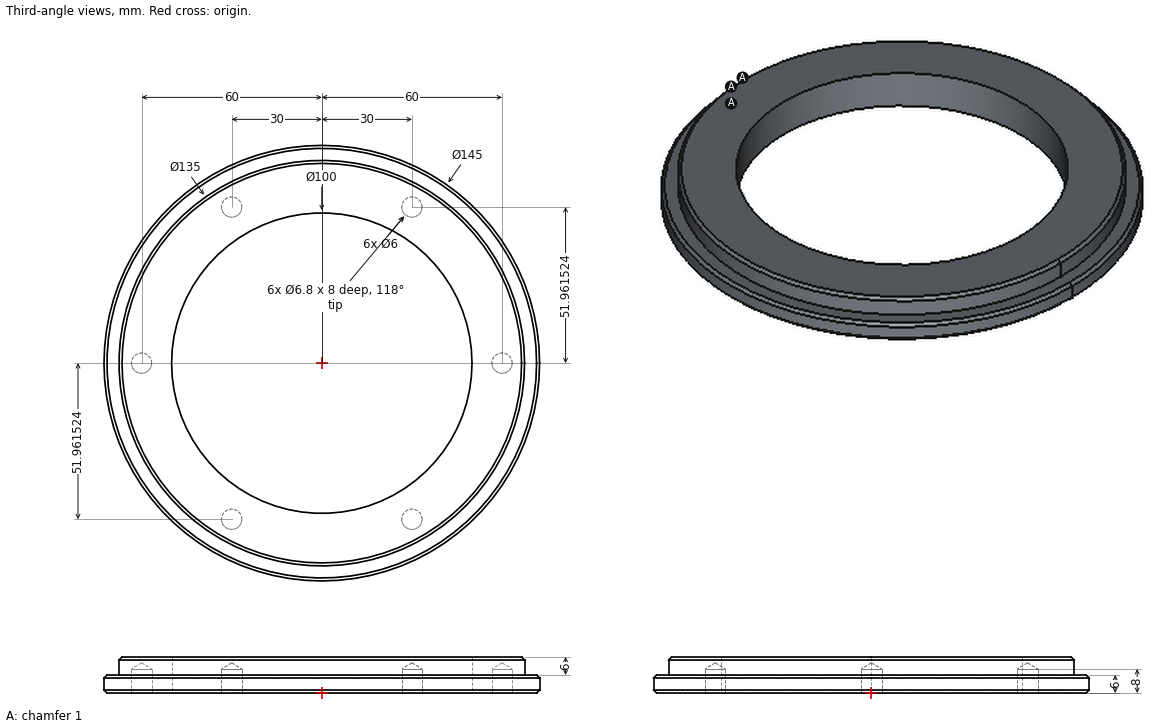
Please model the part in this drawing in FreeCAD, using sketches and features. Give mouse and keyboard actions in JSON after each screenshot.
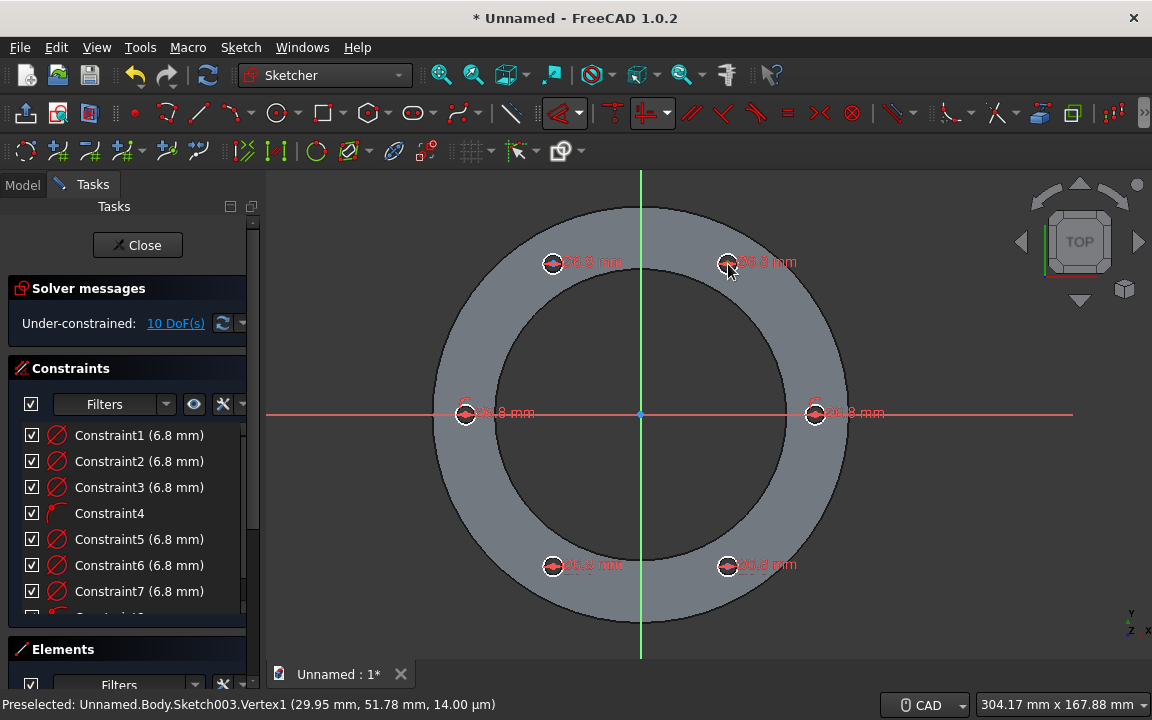
{"action": "left_click", "coordinate": [553, 264]}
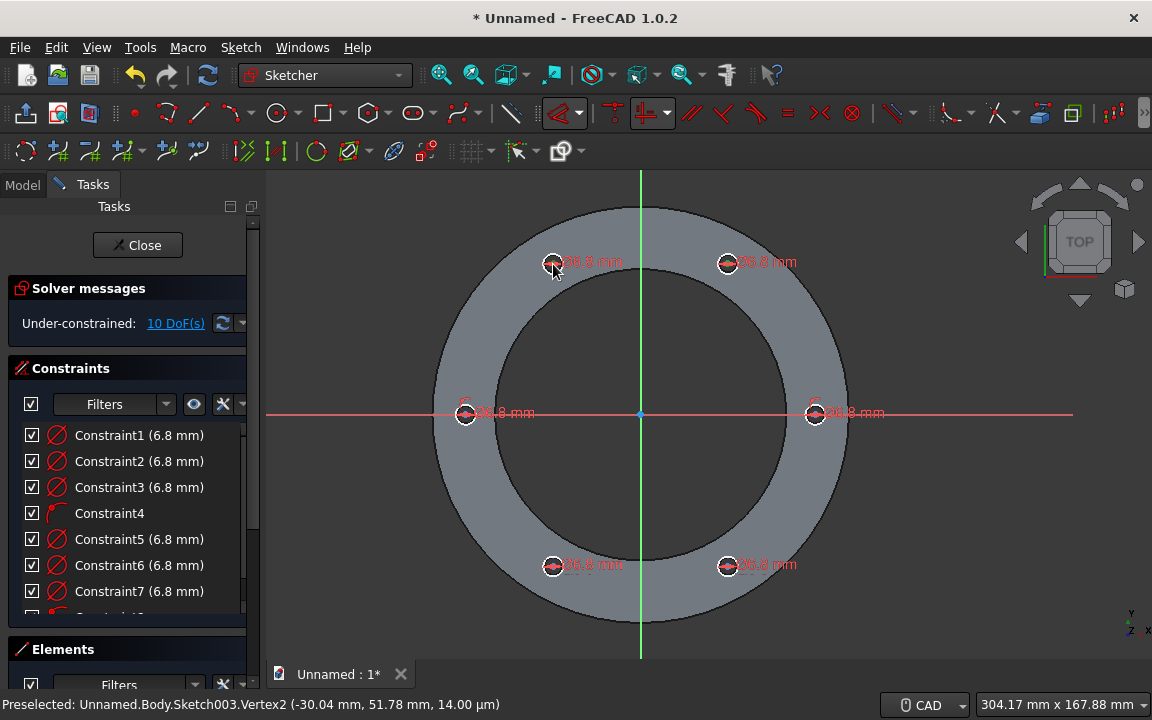
{"action": "left_click", "coordinate": [670, 114]}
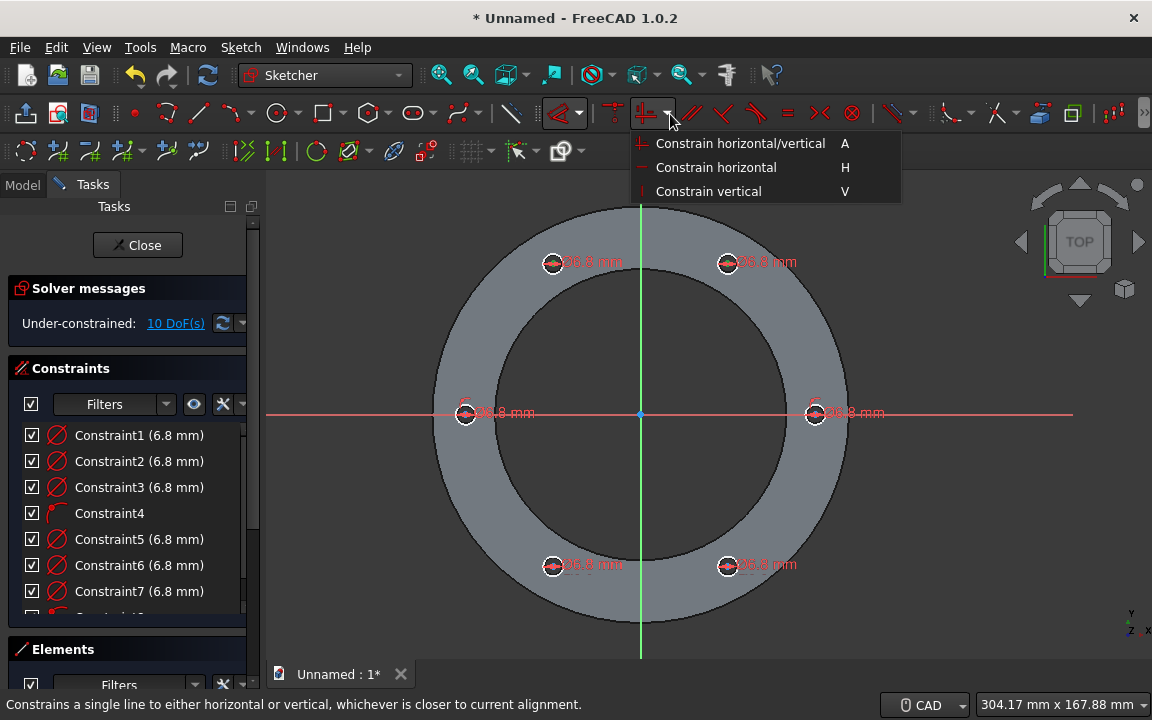
{"action": "left_click", "coordinate": [766, 167]}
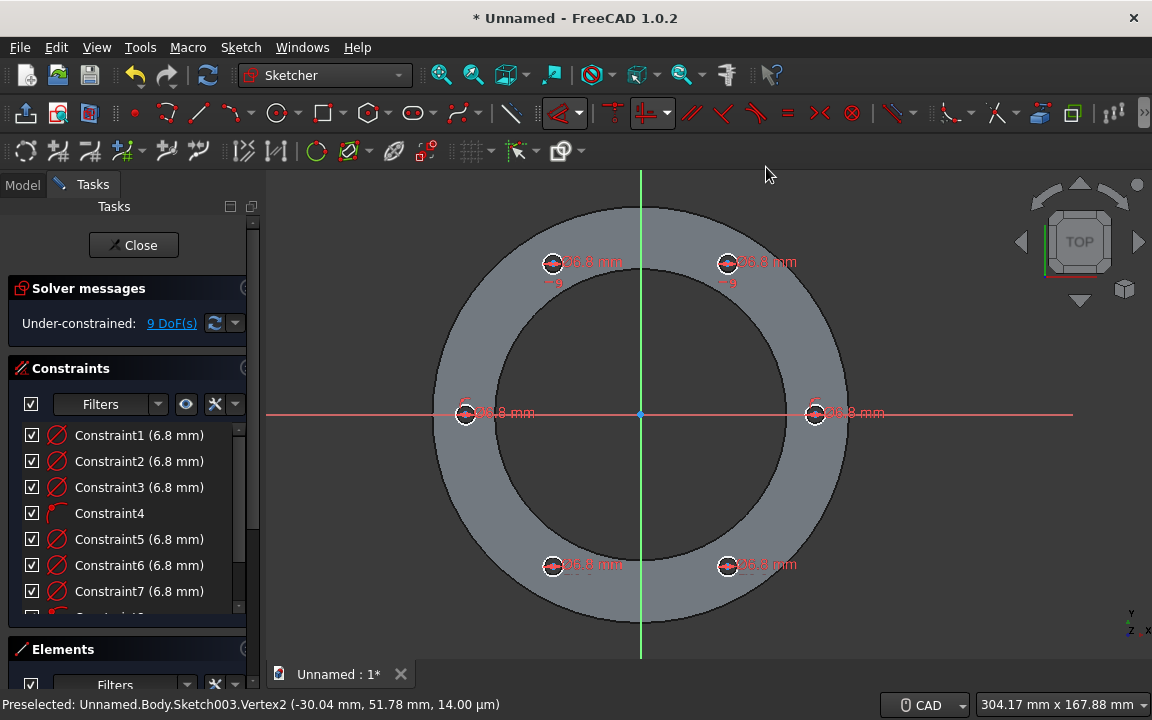
{"action": "left_click", "coordinate": [553, 264]}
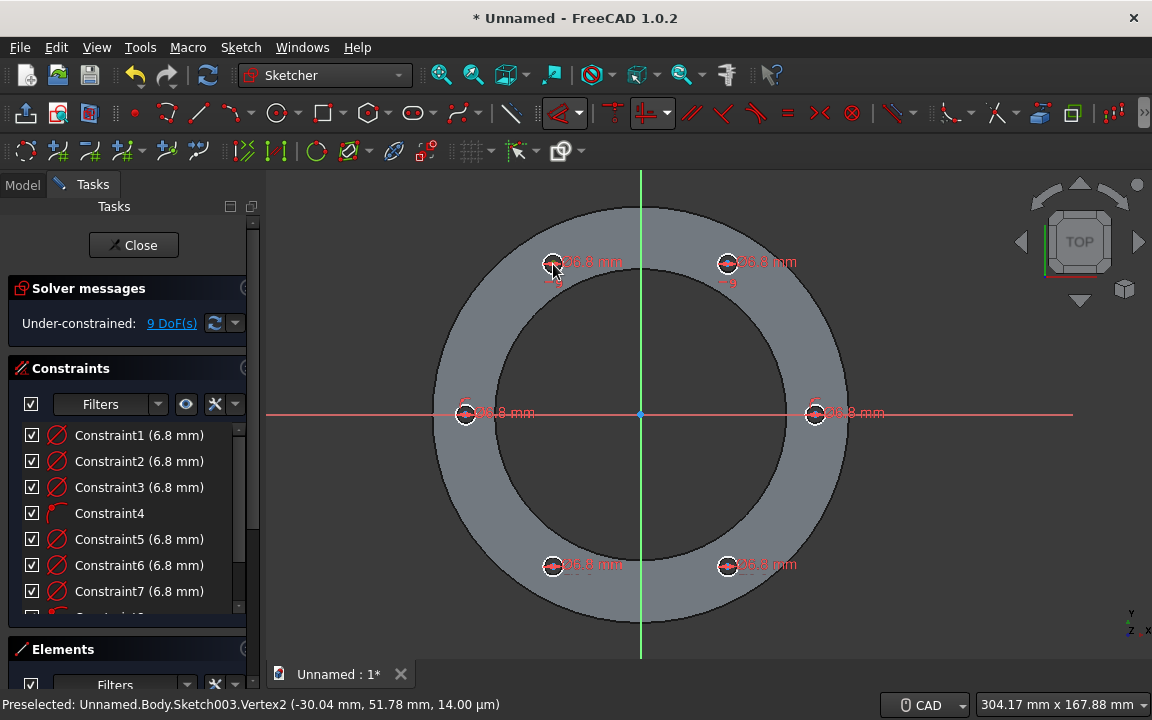
{"action": "left_click", "coordinate": [553, 567]}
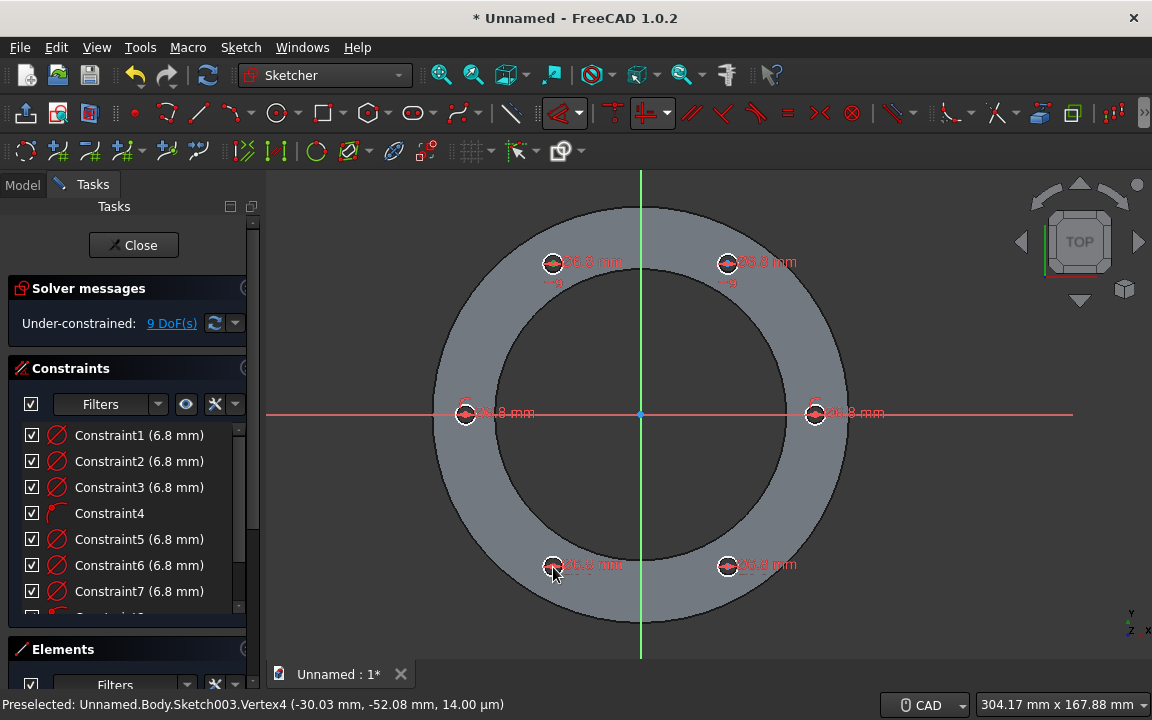
{"action": "left_click", "coordinate": [670, 114]}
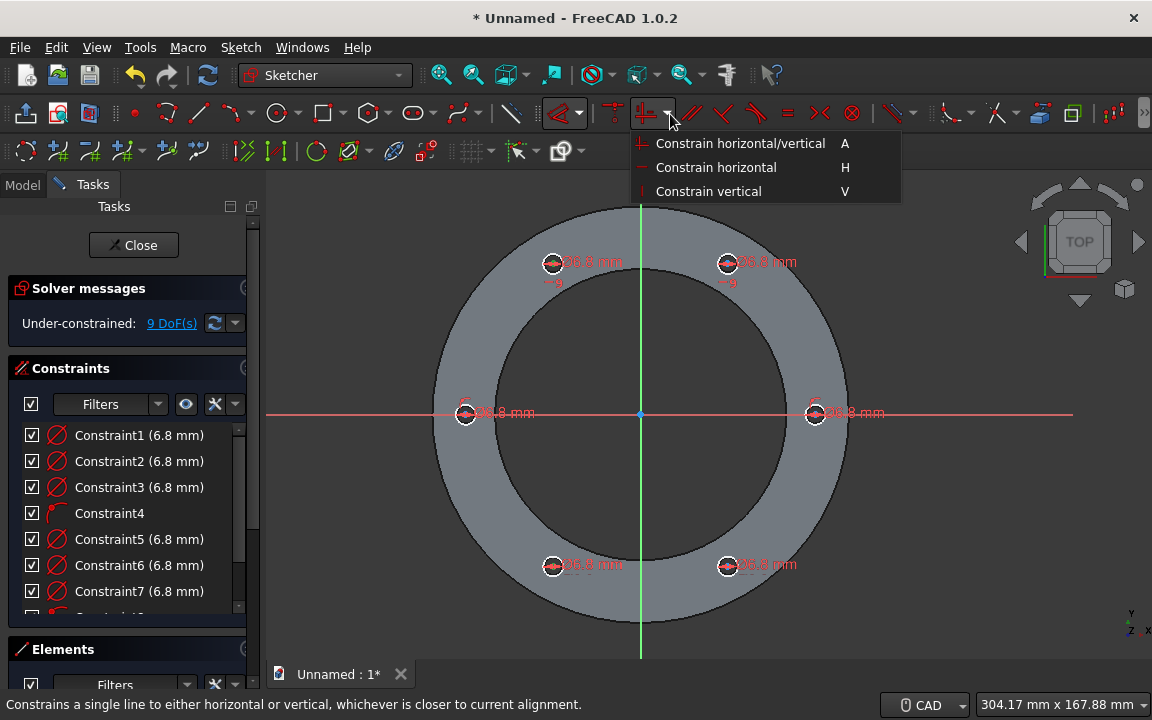
{"action": "left_click", "coordinate": [766, 191]}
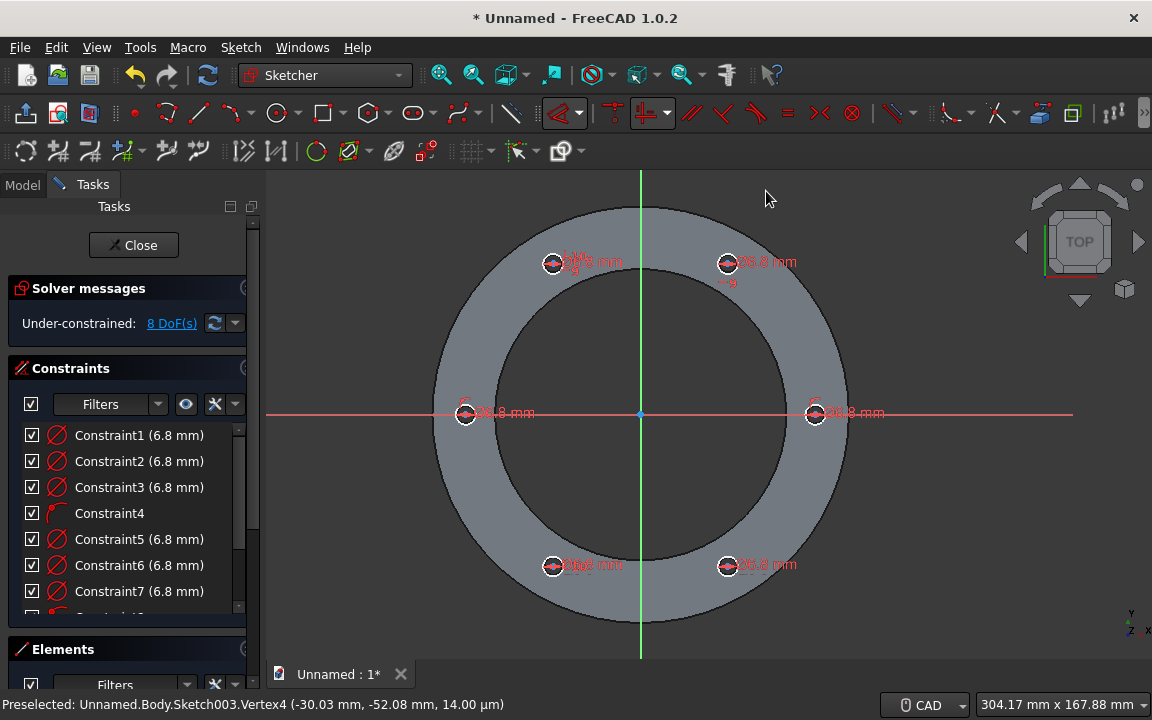
{"action": "left_click", "coordinate": [728, 264]}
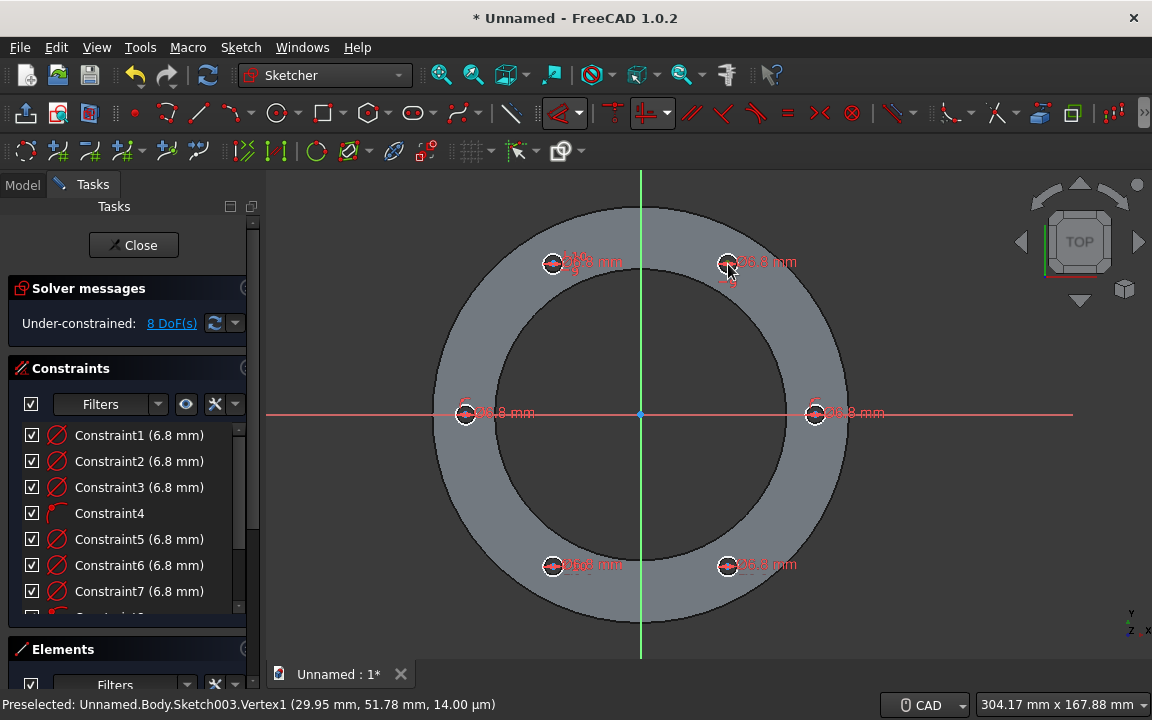
{"action": "left_click", "coordinate": [728, 567]}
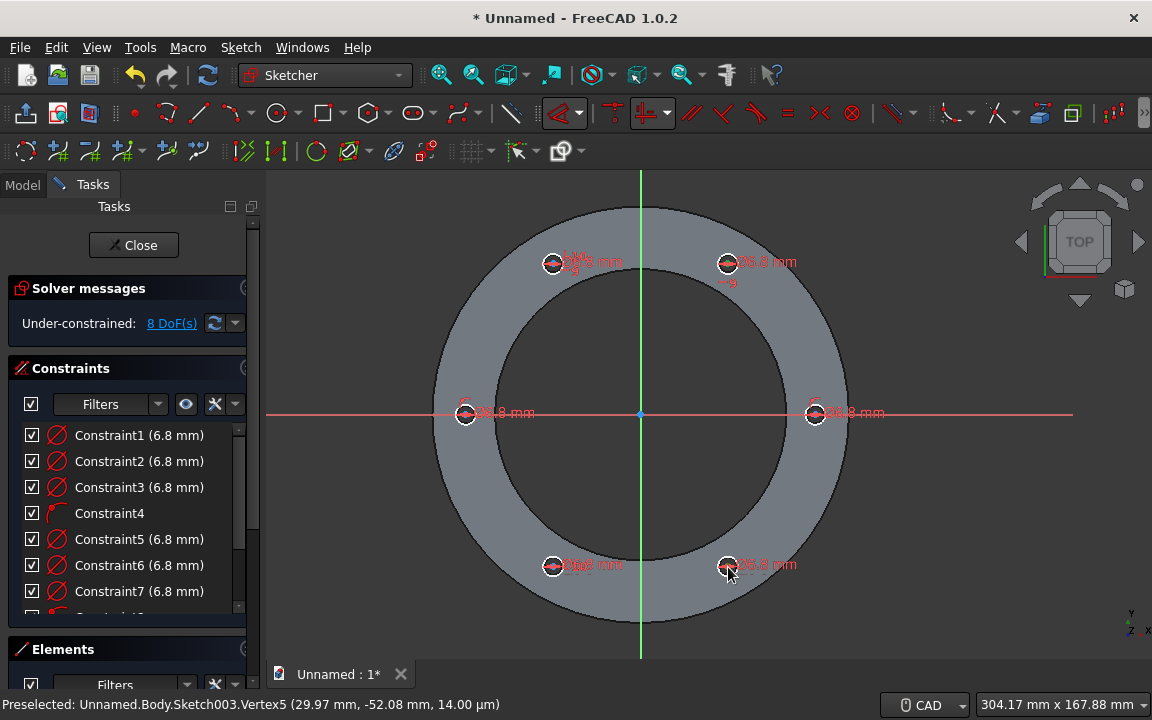
{"action": "left_click", "coordinate": [670, 114]}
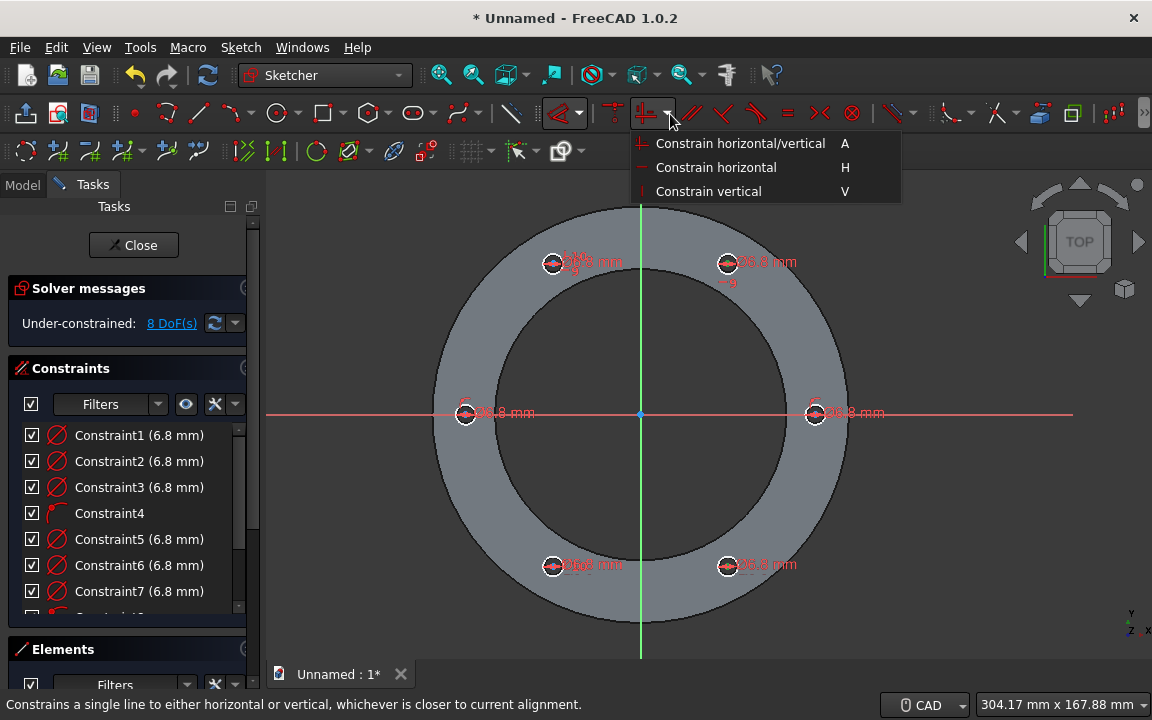
{"action": "left_click", "coordinate": [766, 191]}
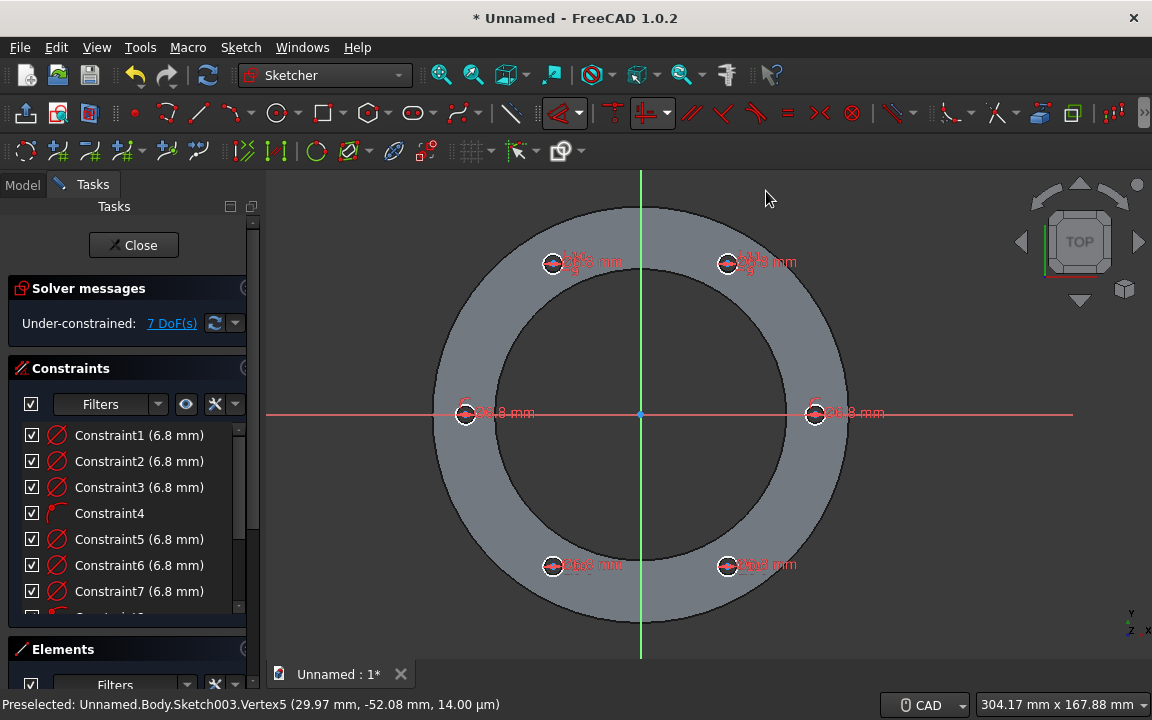
{"action": "left_click", "coordinate": [553, 567]}